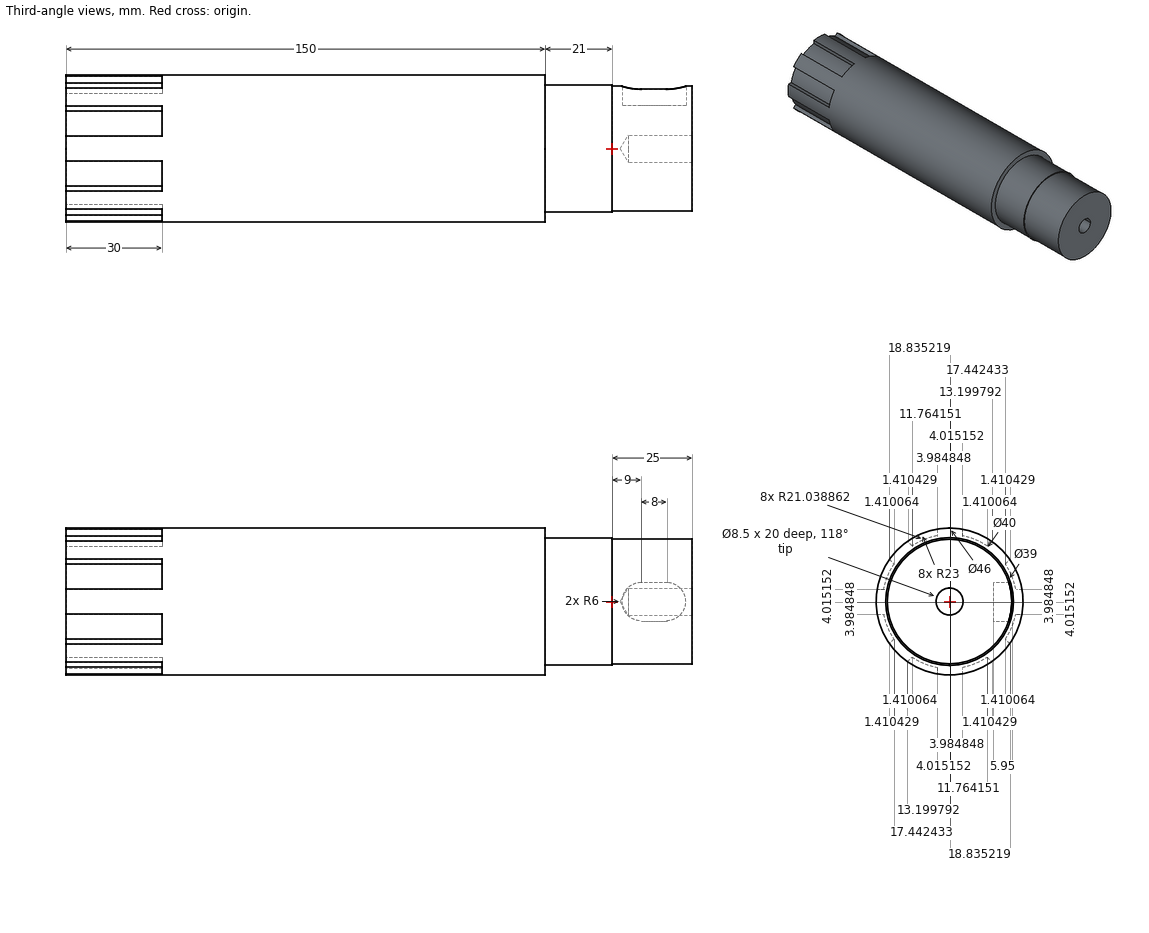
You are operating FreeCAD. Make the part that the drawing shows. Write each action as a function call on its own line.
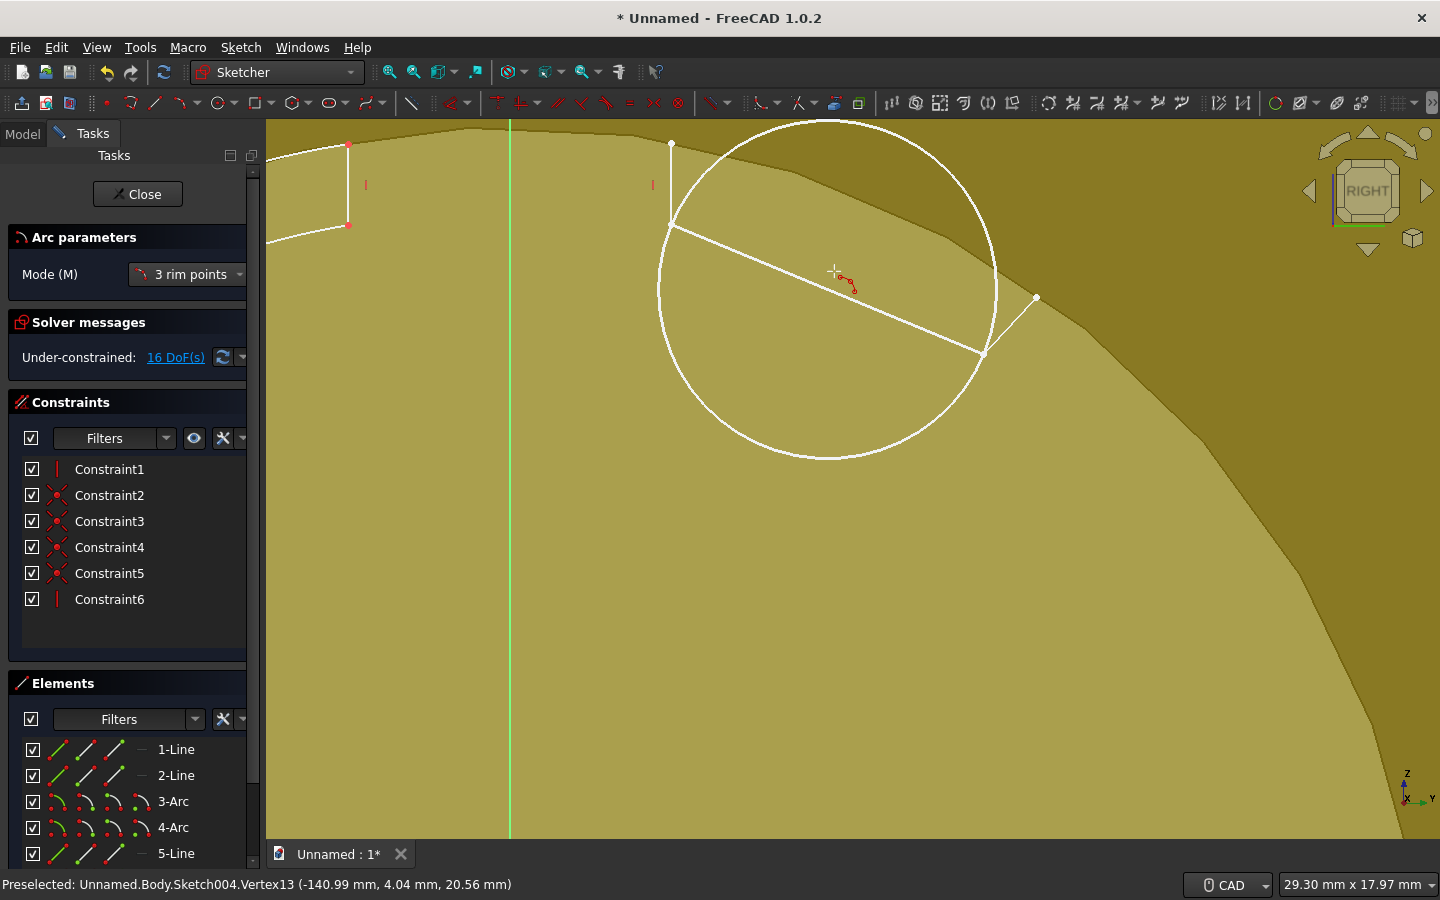
click(833, 270)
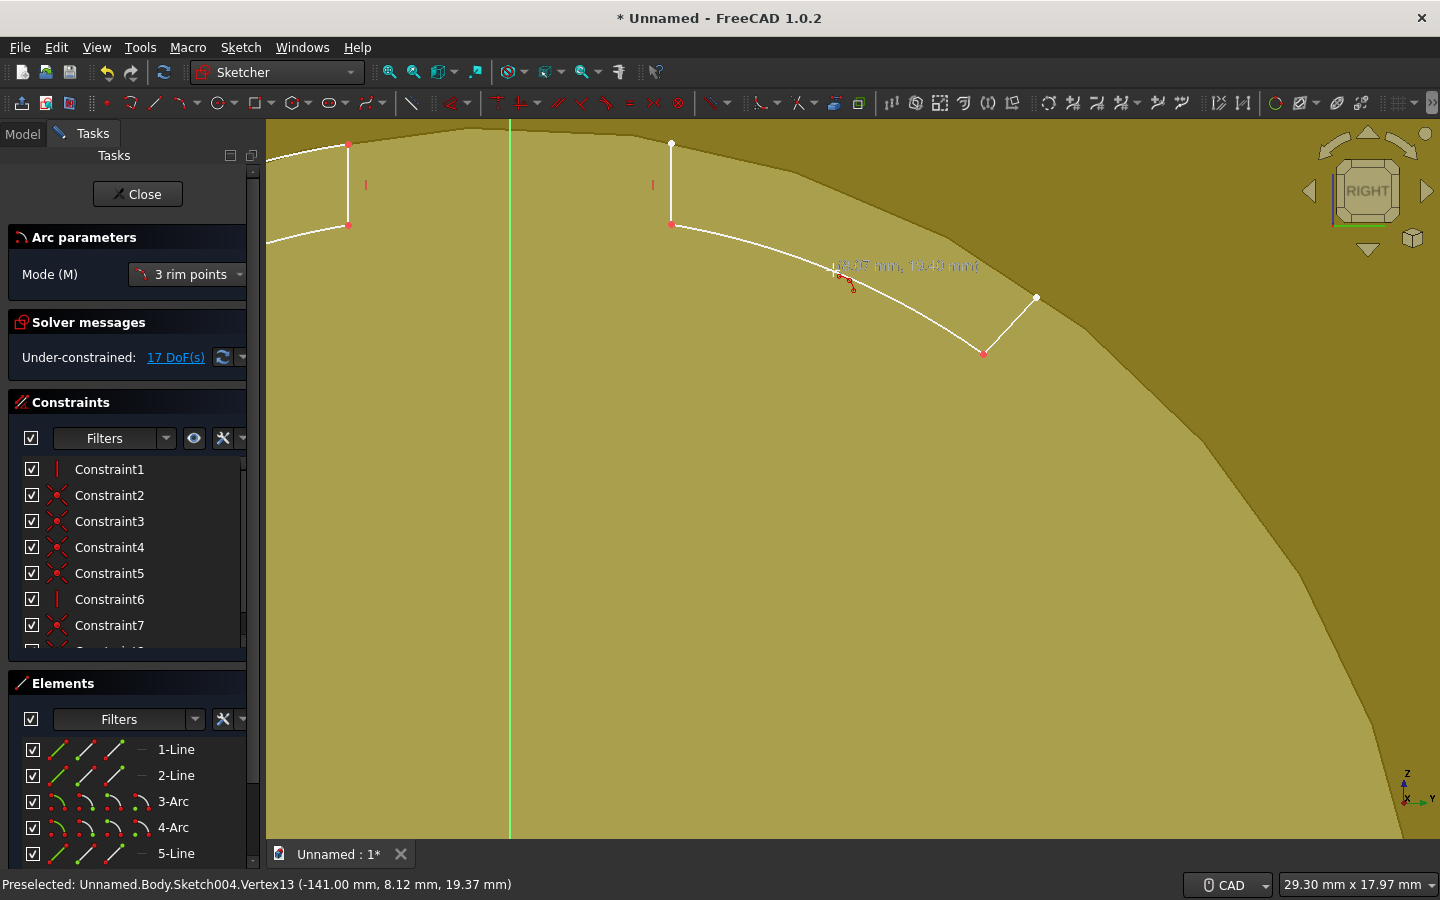
scroll(874, 293, down, 7)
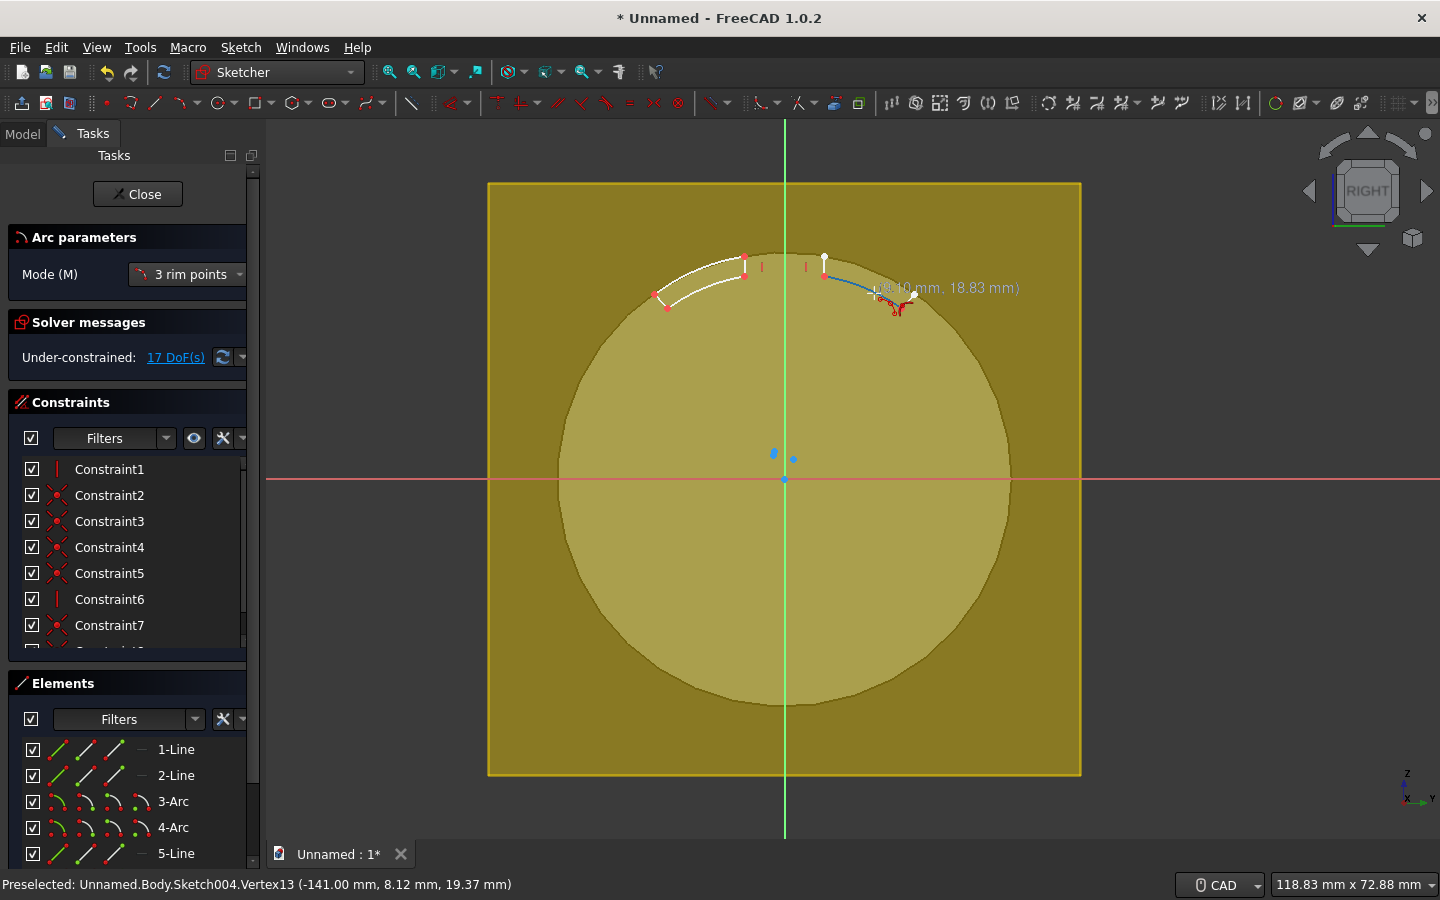
scroll(824, 256, up, 3)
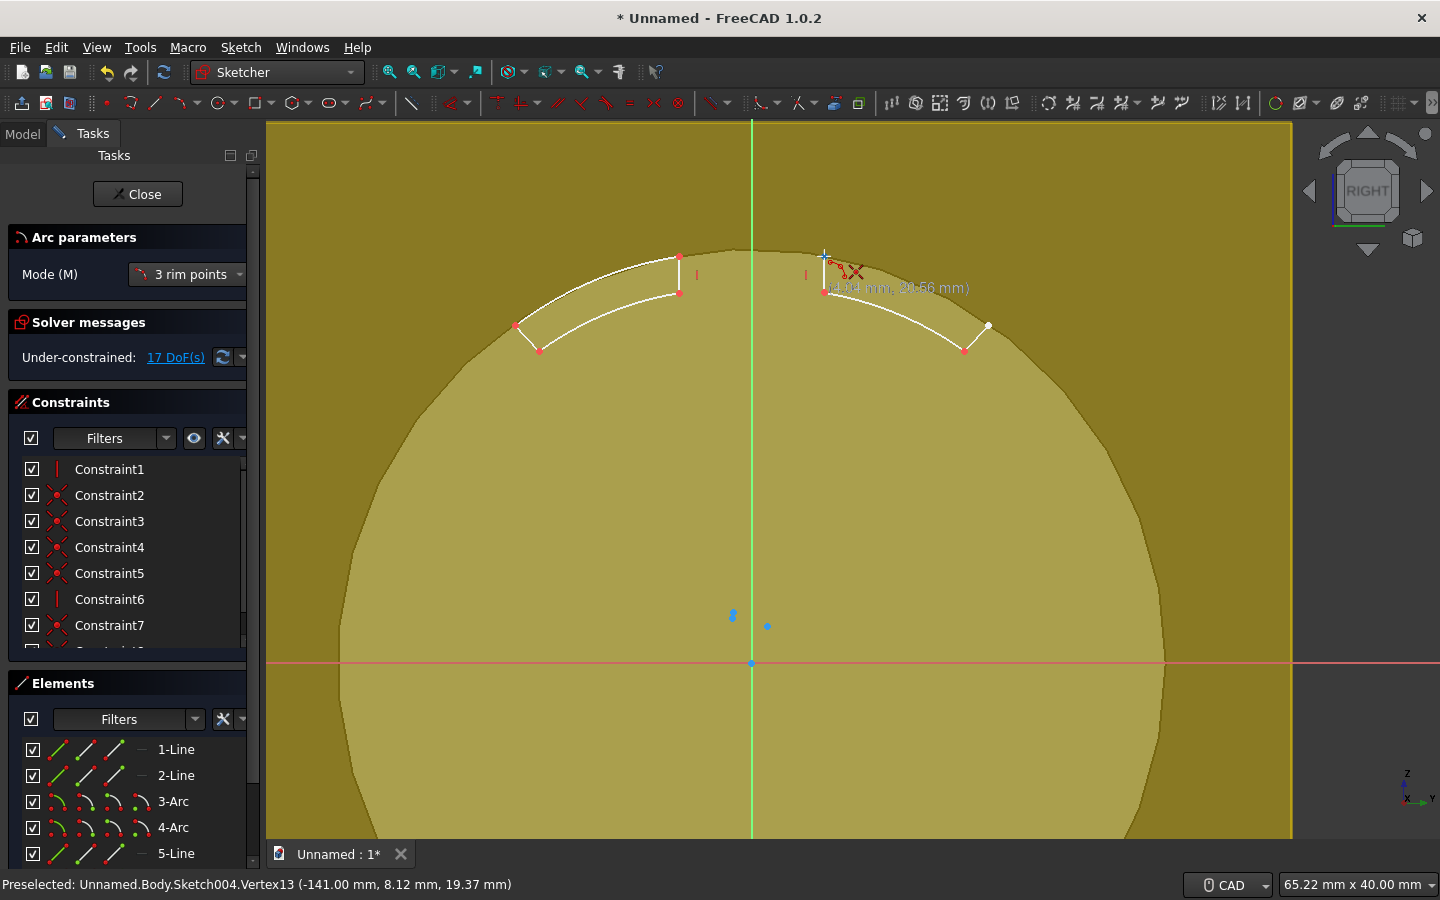
click(824, 256)
click(988, 326)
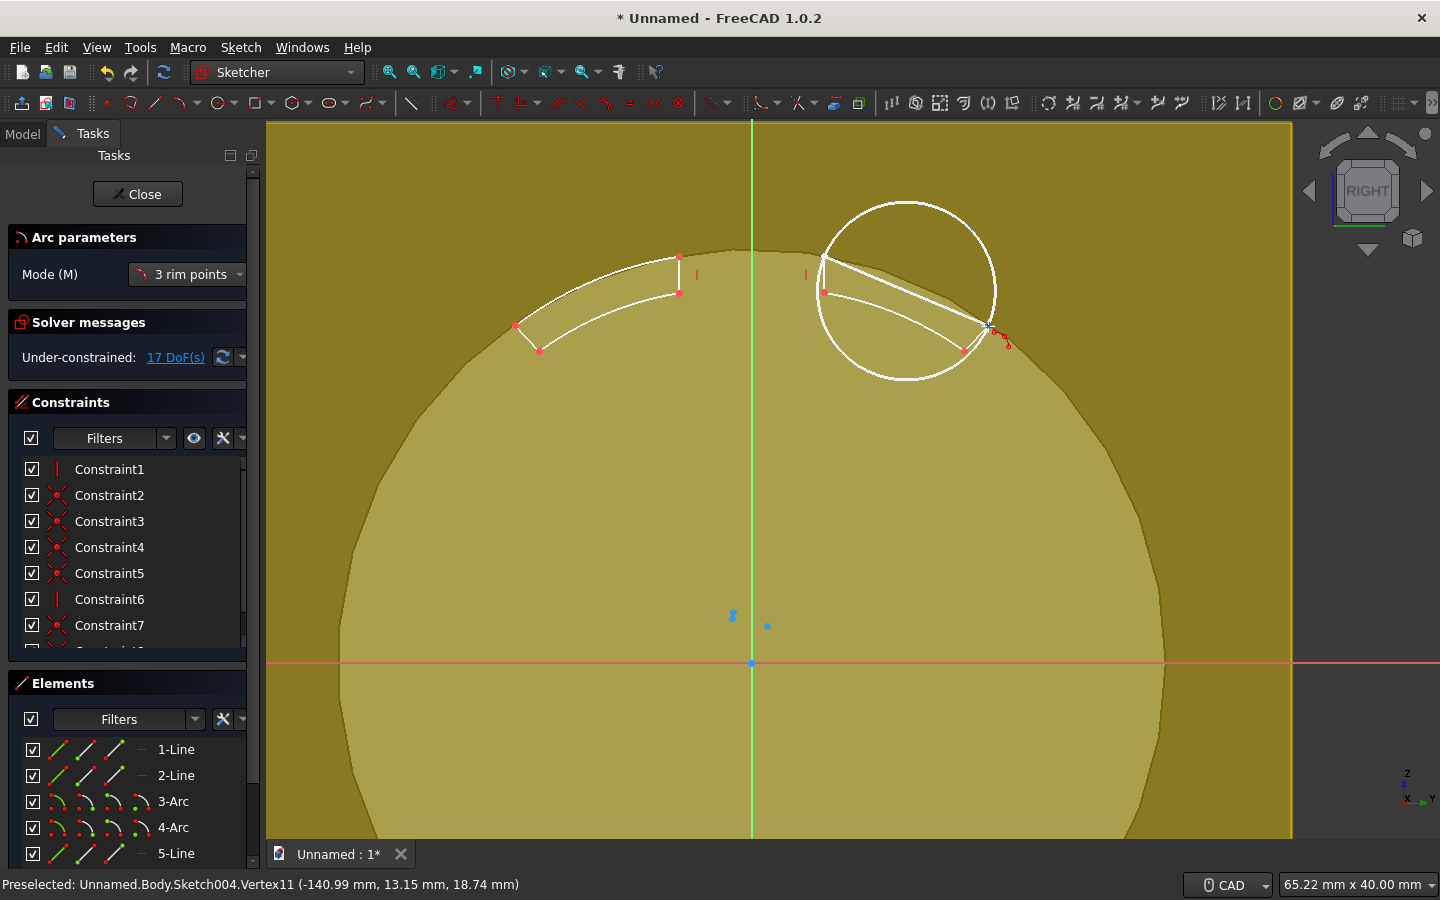
scroll(910, 281, up, 3)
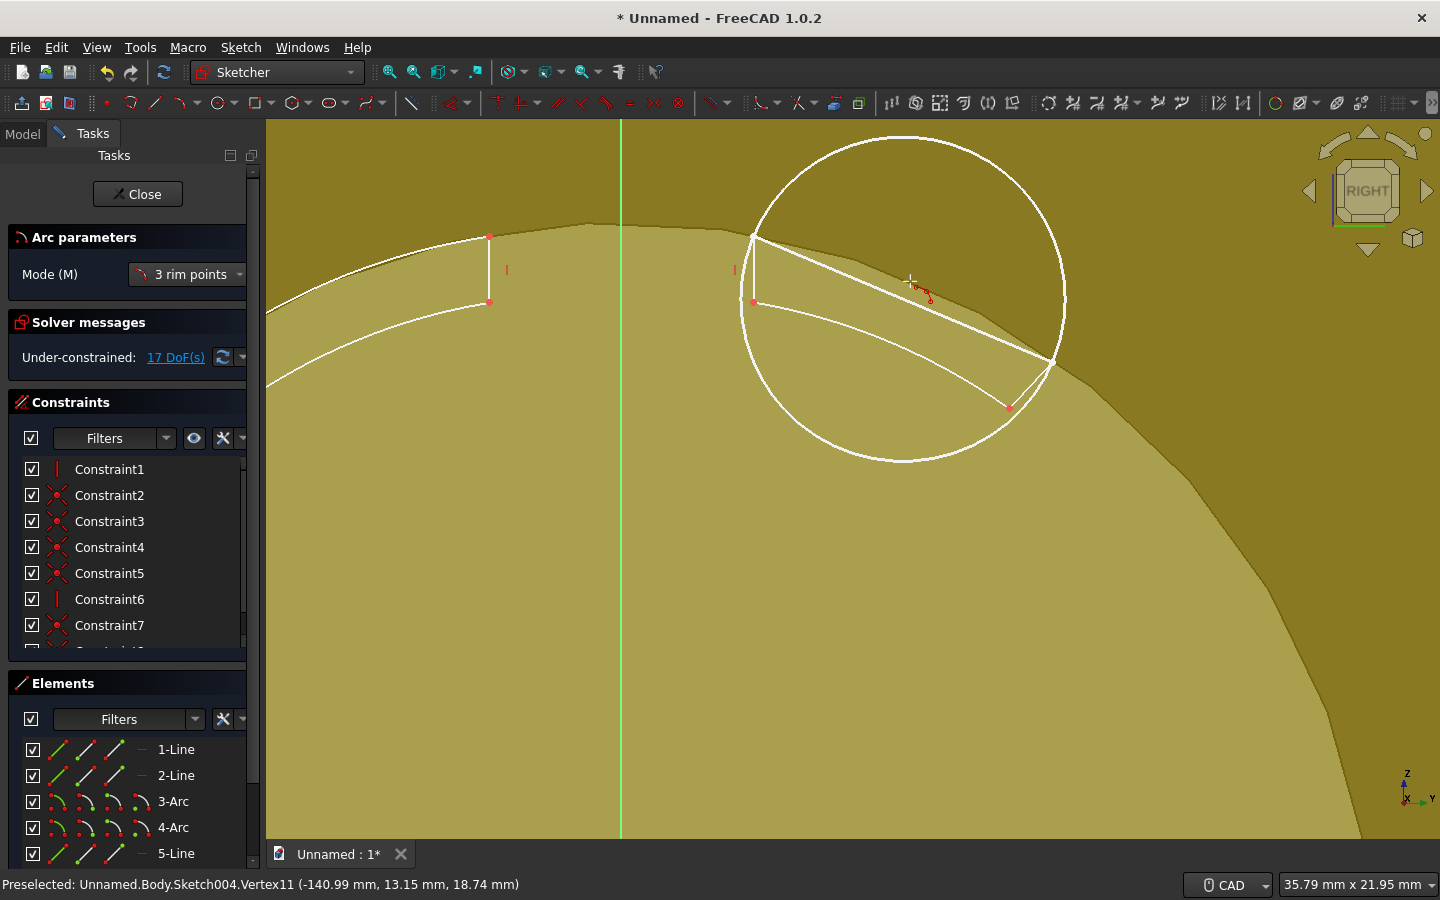
click(910, 280)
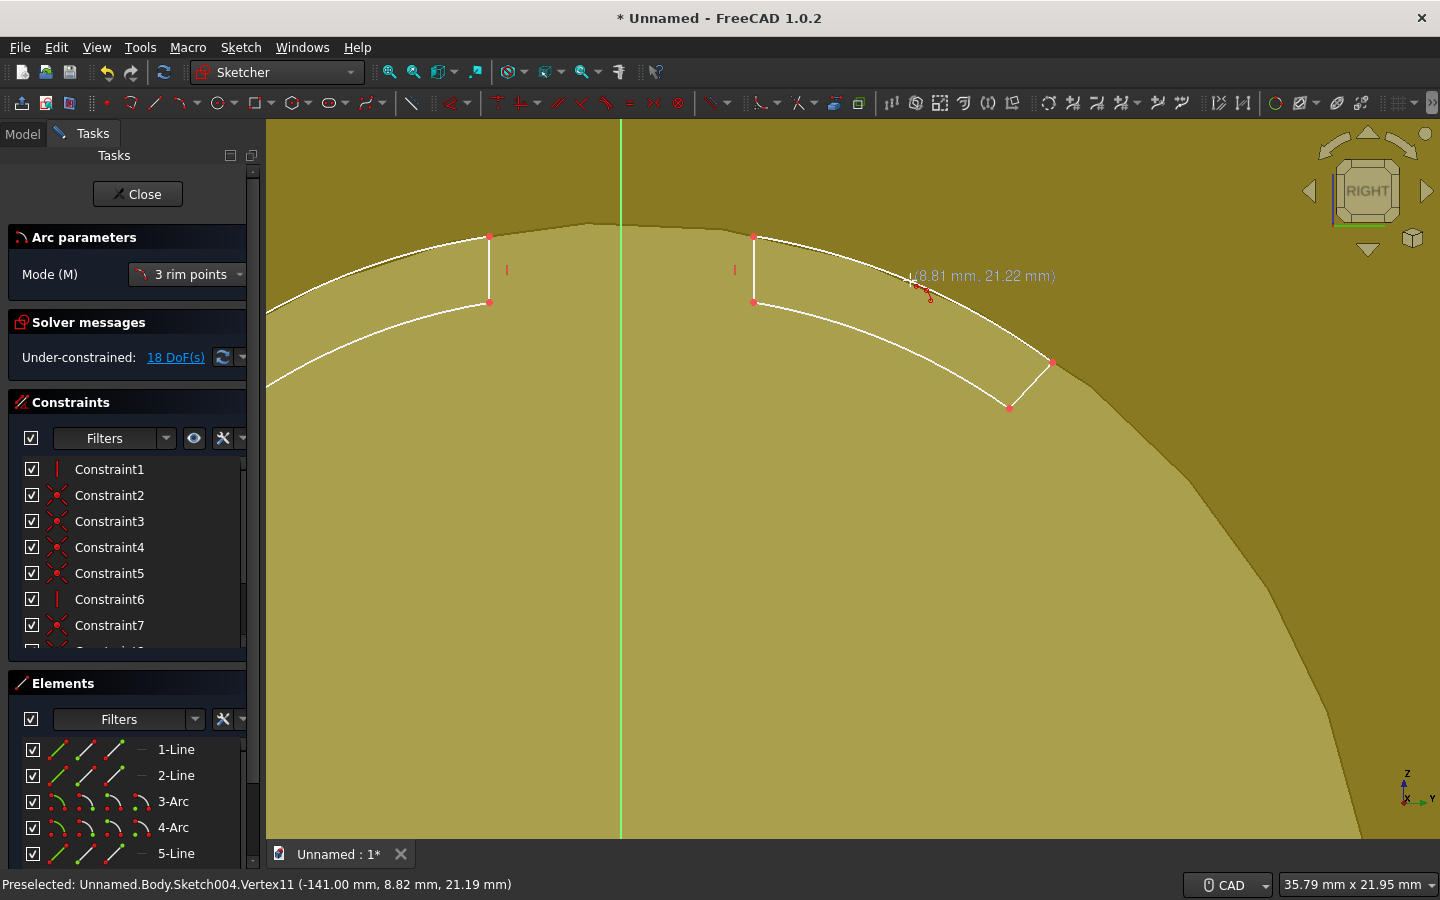
click(156, 104)